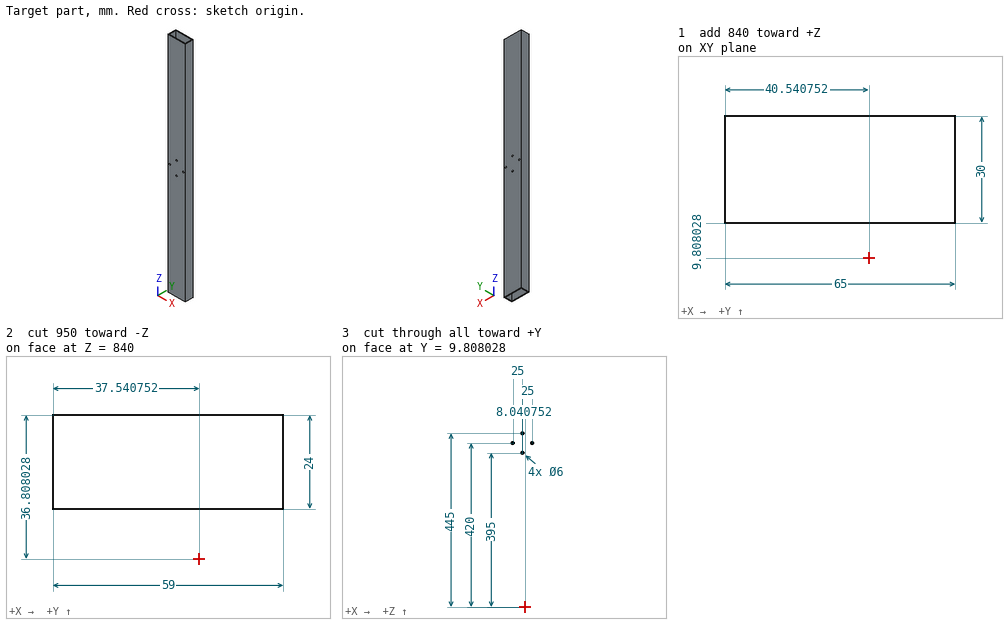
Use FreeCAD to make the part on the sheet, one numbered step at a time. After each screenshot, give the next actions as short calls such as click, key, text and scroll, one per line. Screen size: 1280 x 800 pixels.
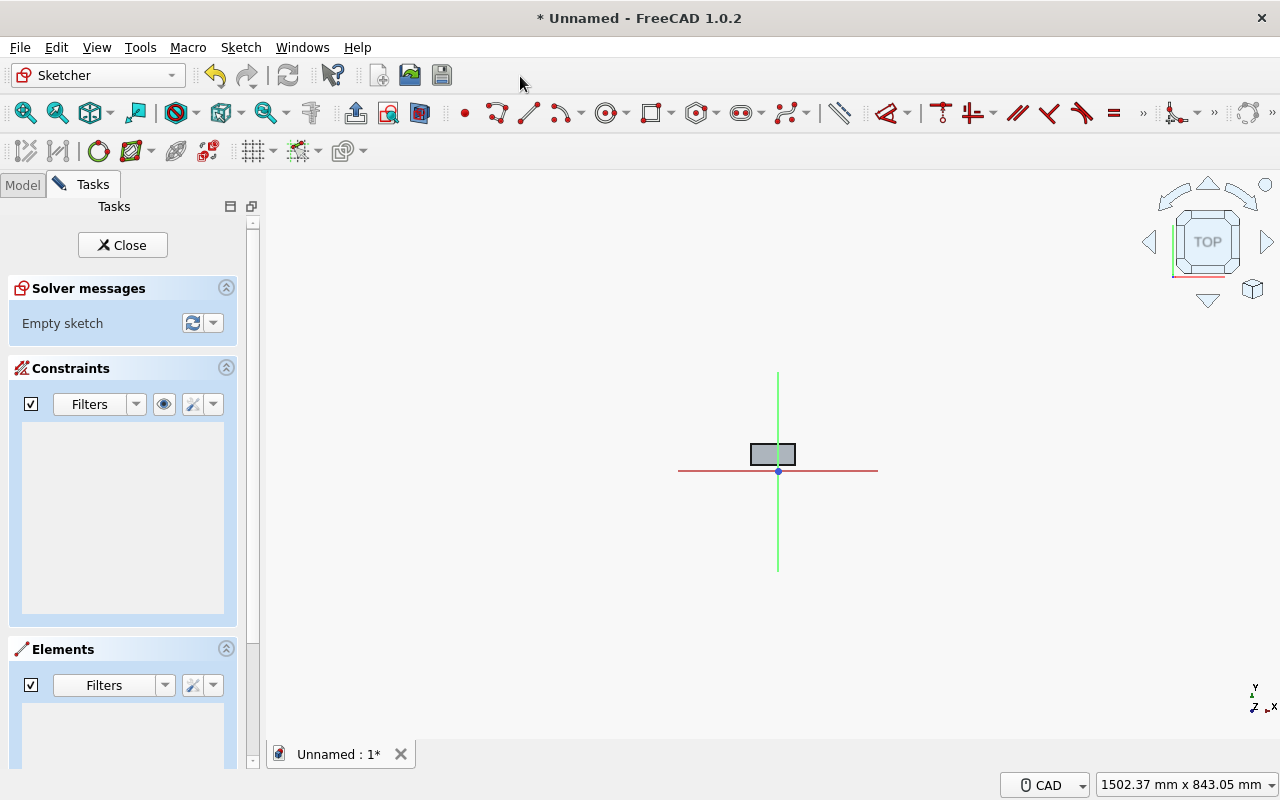
scroll(778, 459, up, 13)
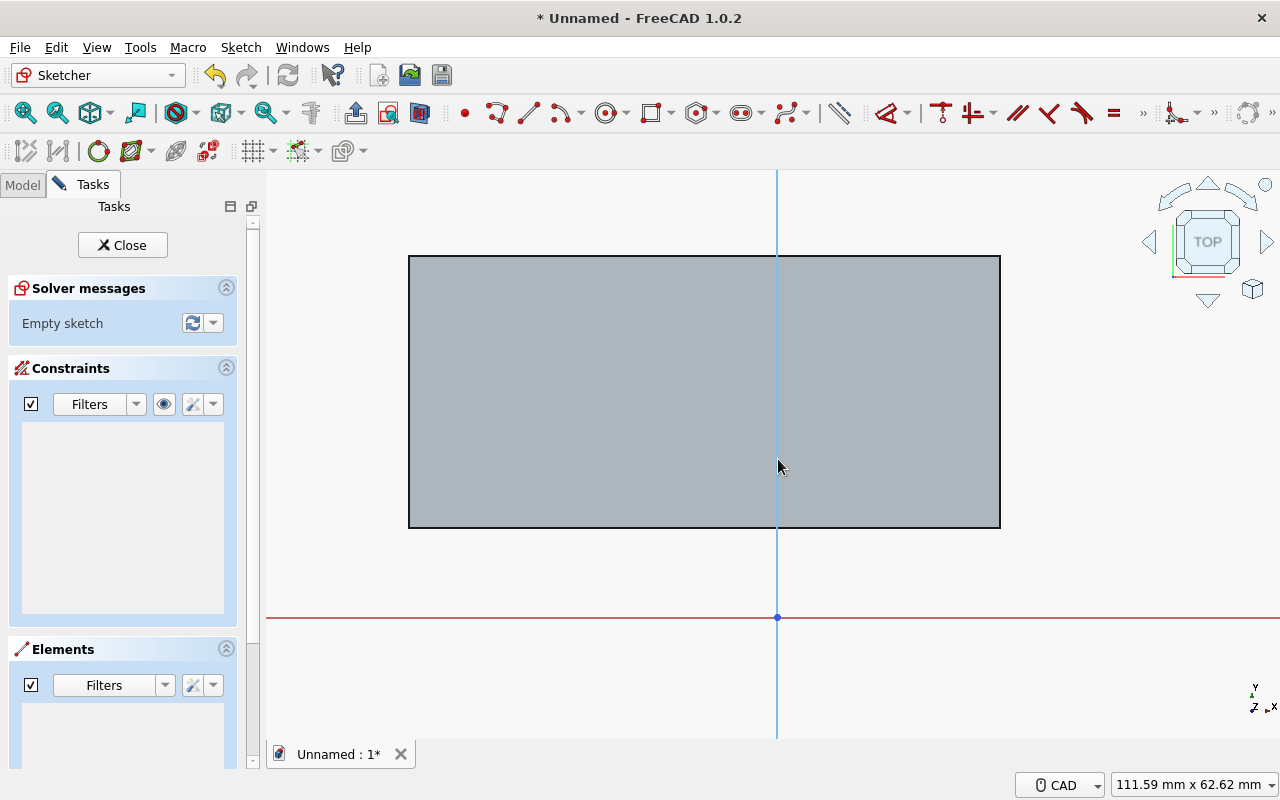
click(652, 114)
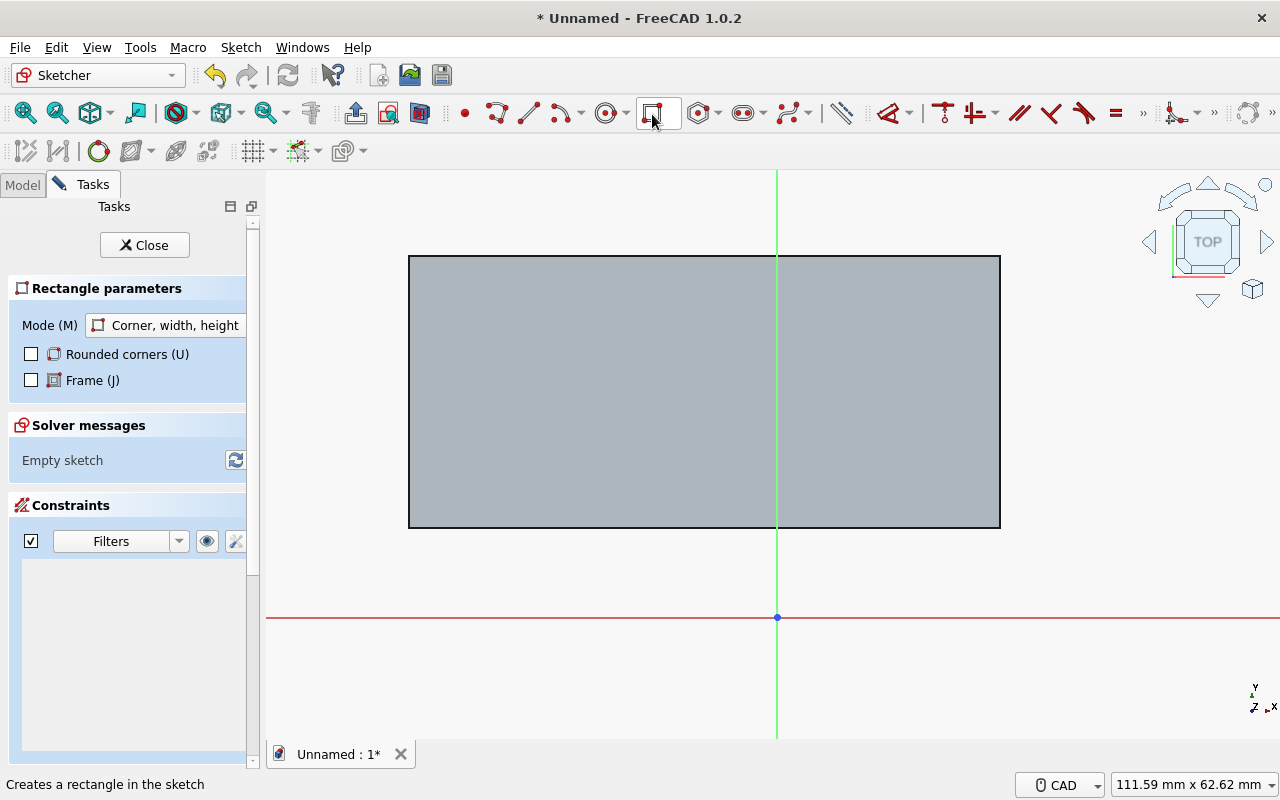
click(436, 283)
move(972, 501)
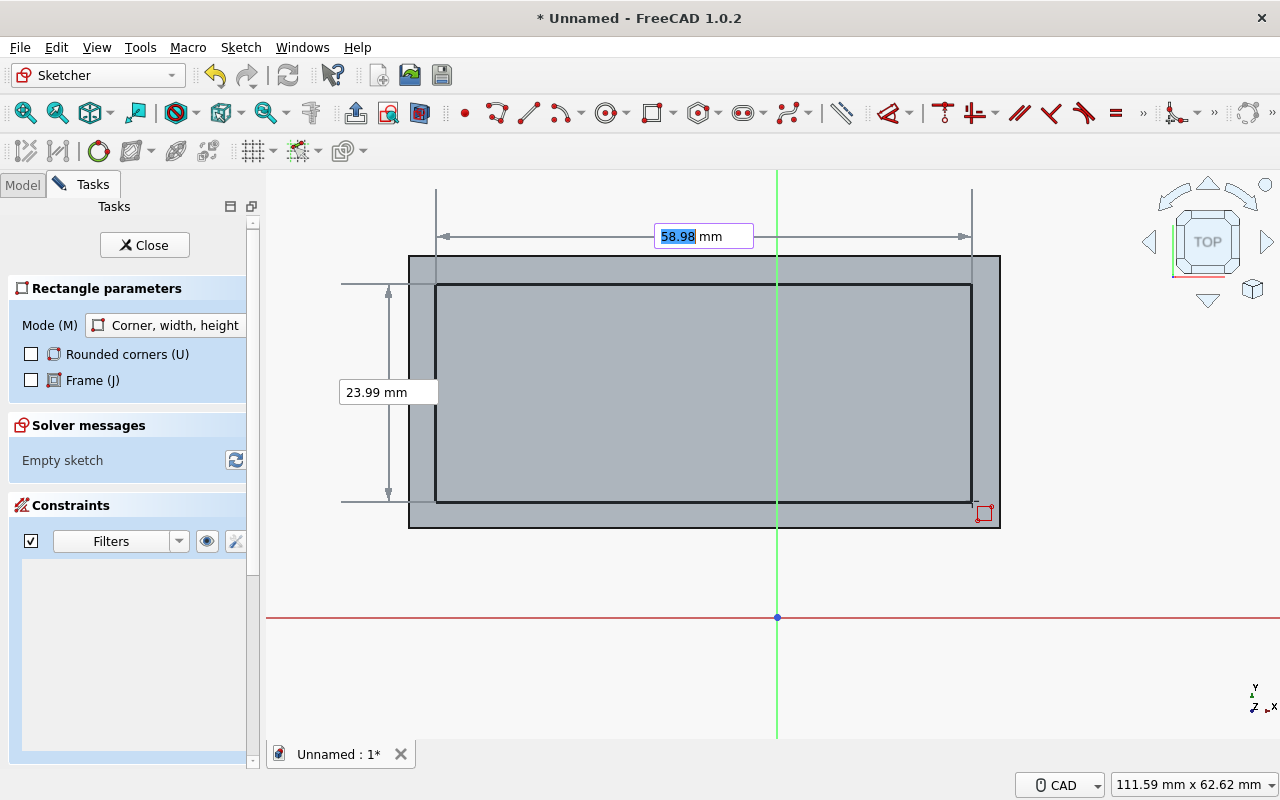
text(59)
key(Tab)
text(24)
key(Return)
key(Escape)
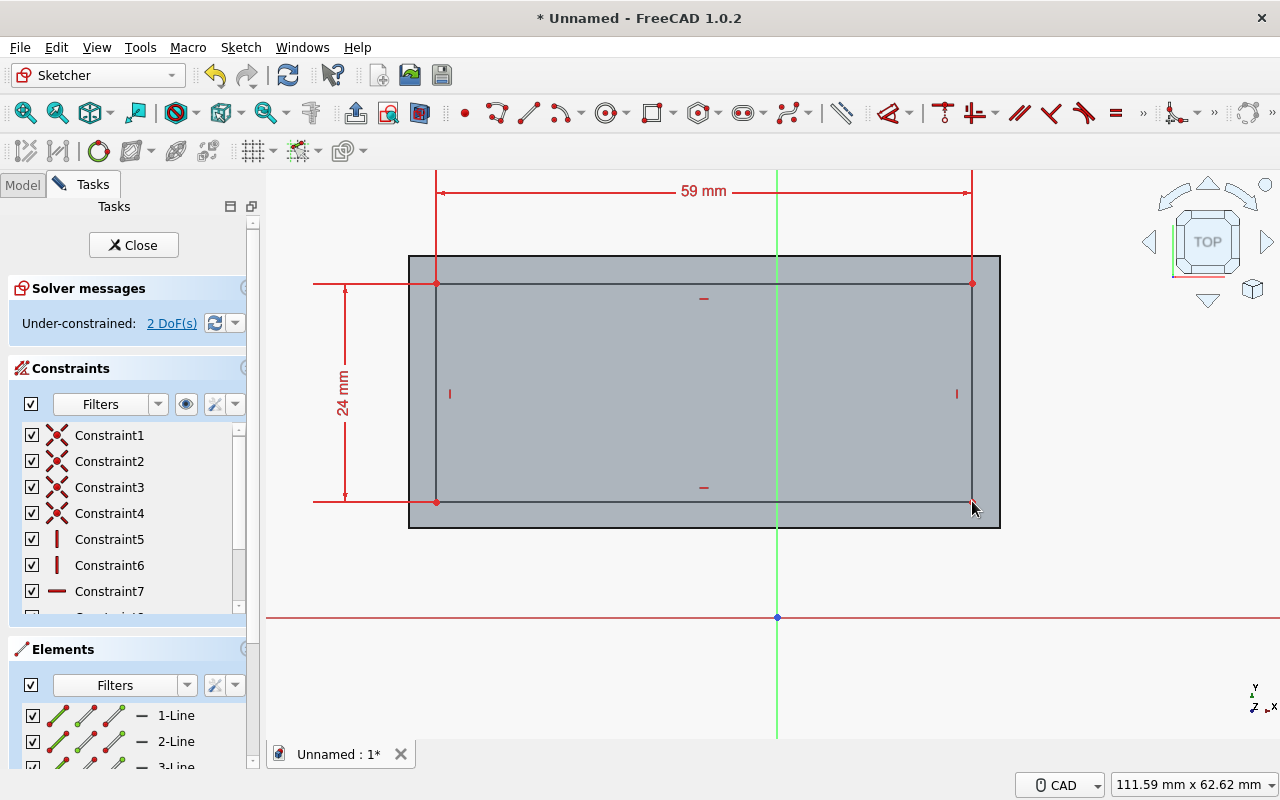
click(888, 114)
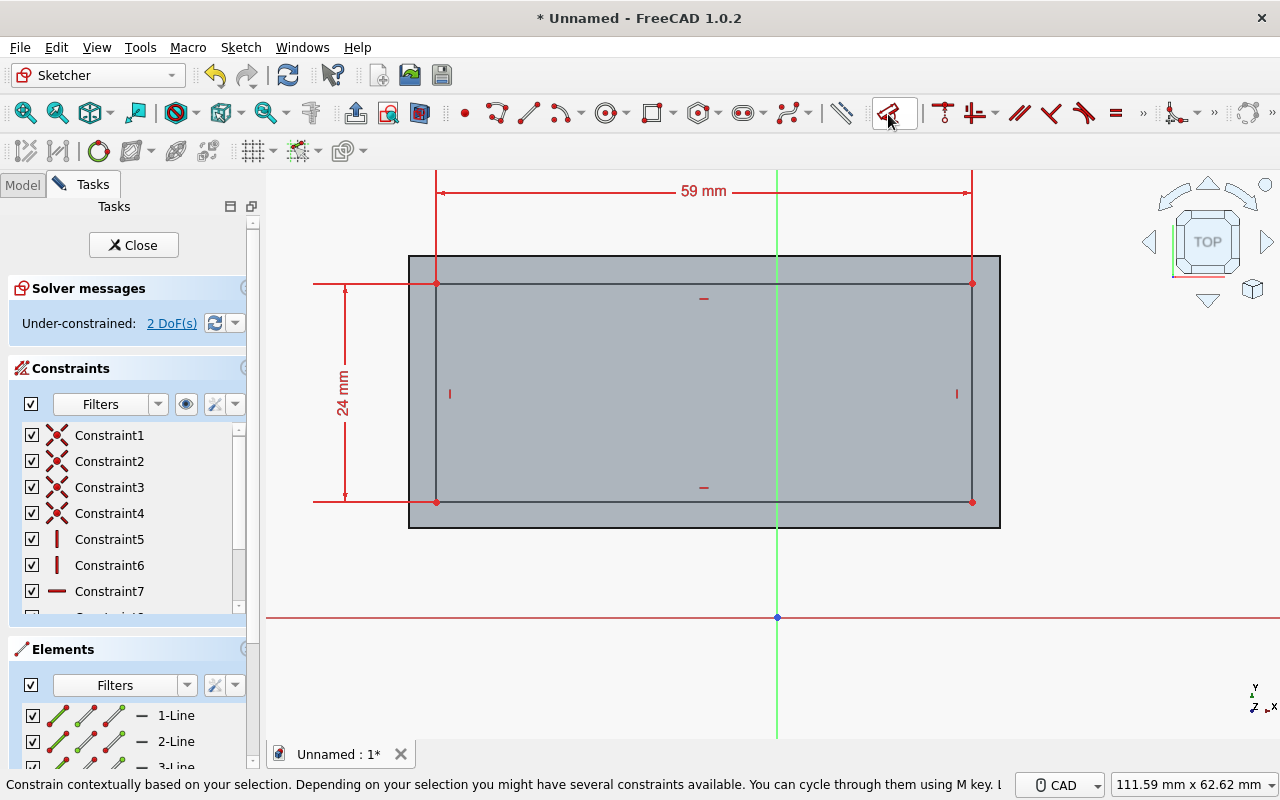
click(436, 284)
click(607, 652)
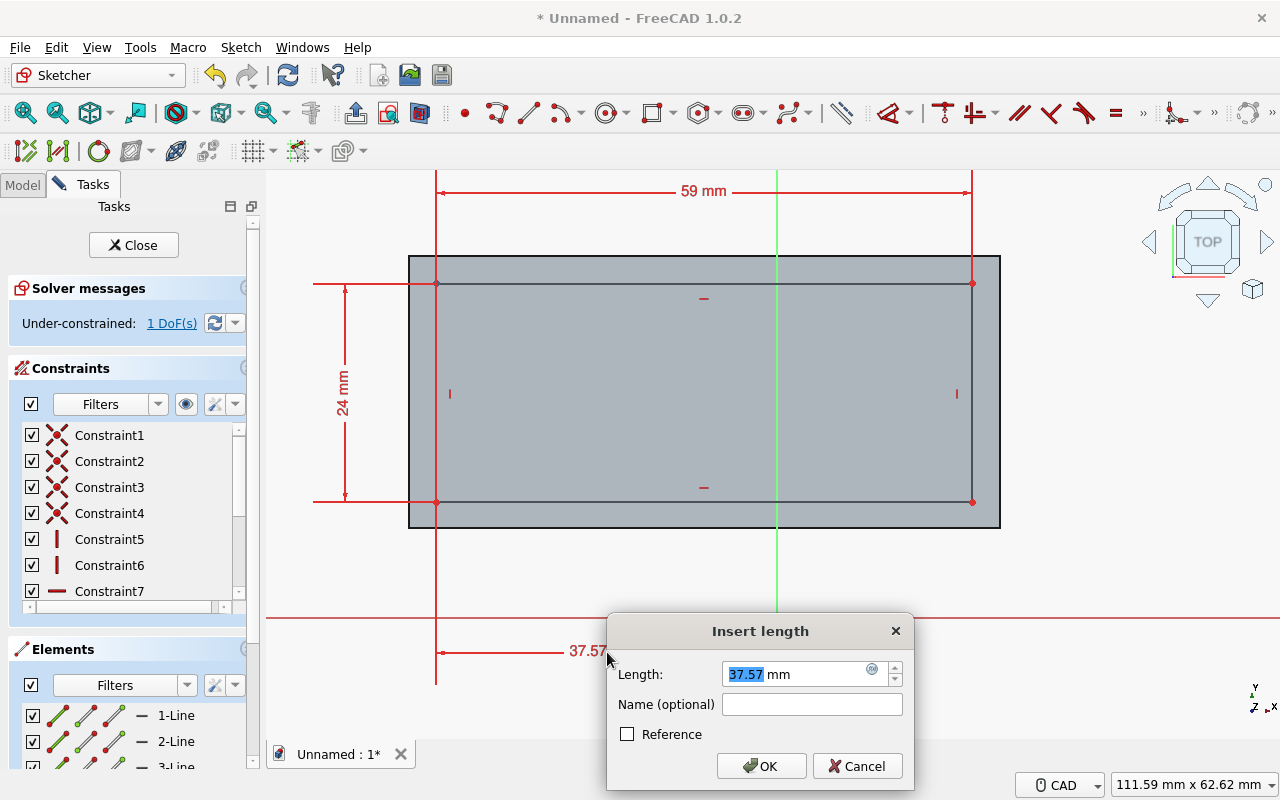
text(37.540752)
key(Return)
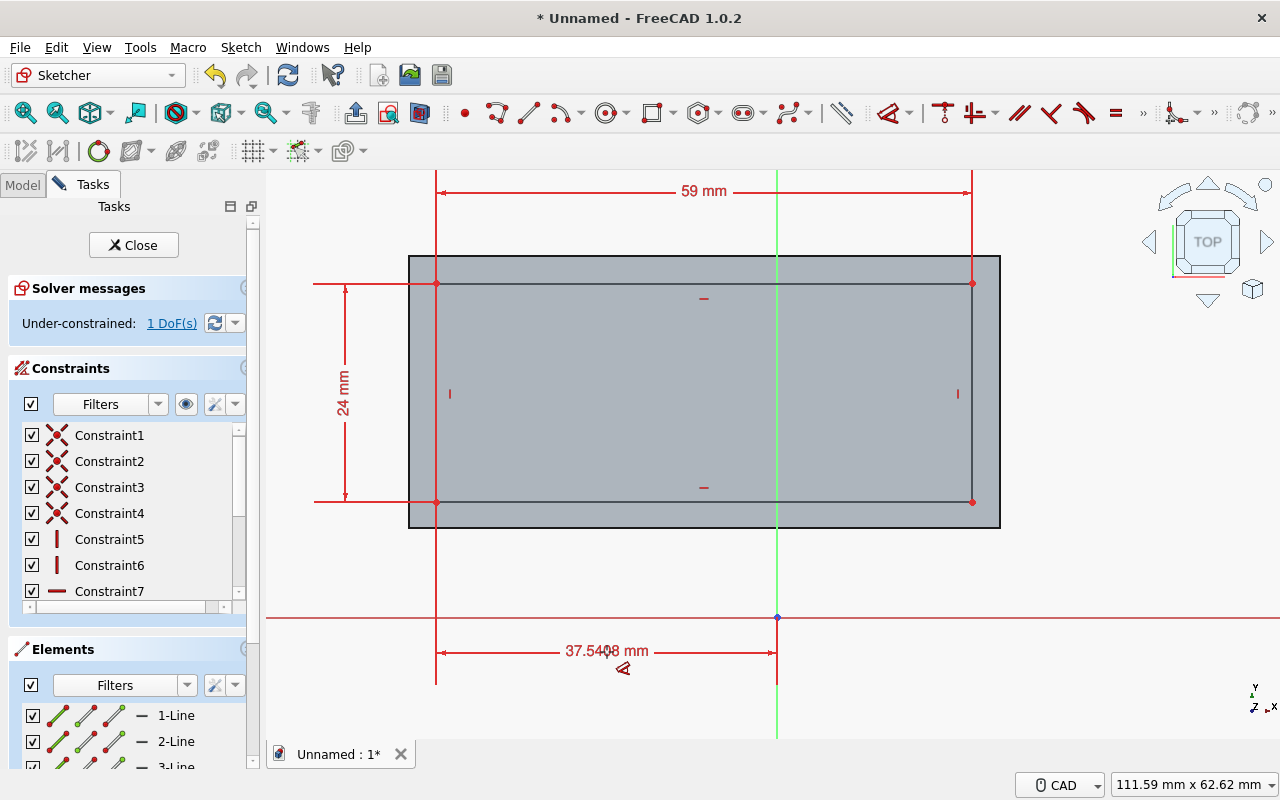
click(436, 284)
click(402, 451)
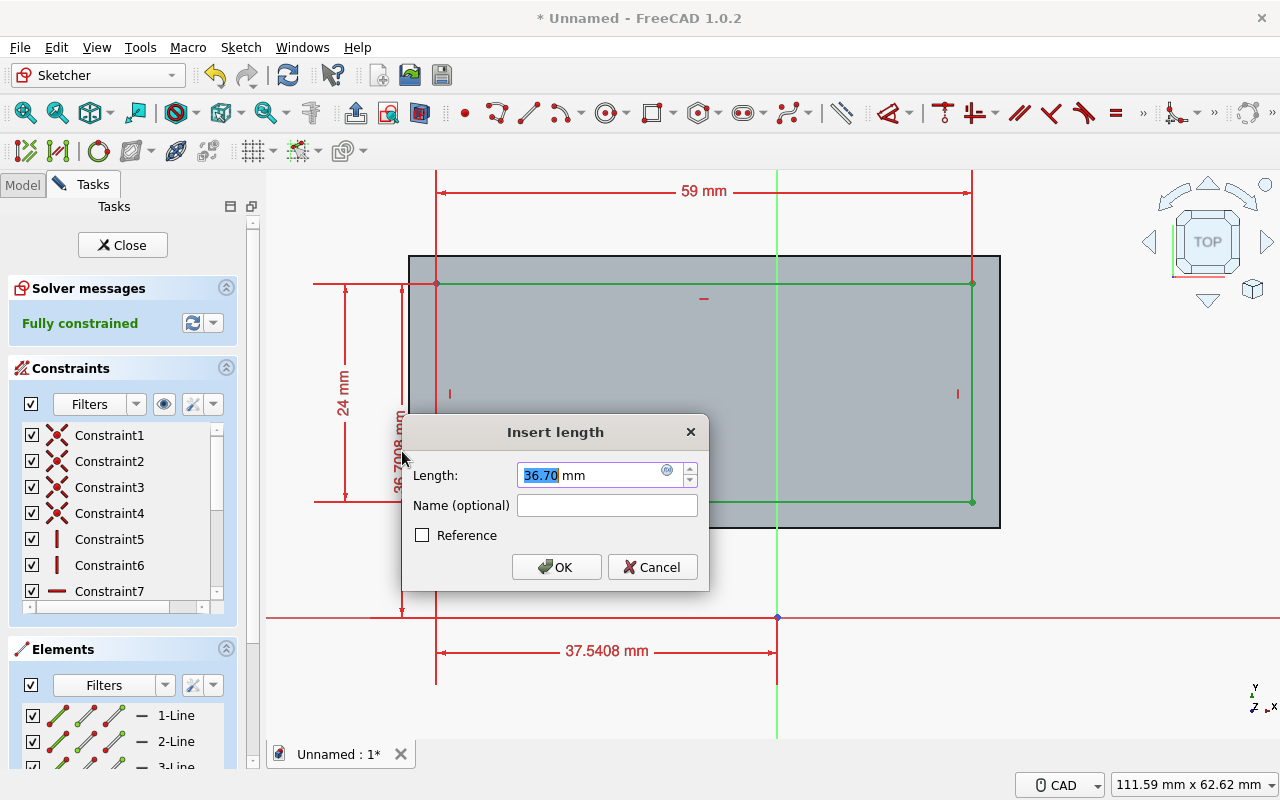
text(36.808028)
key(Return)
key(Escape)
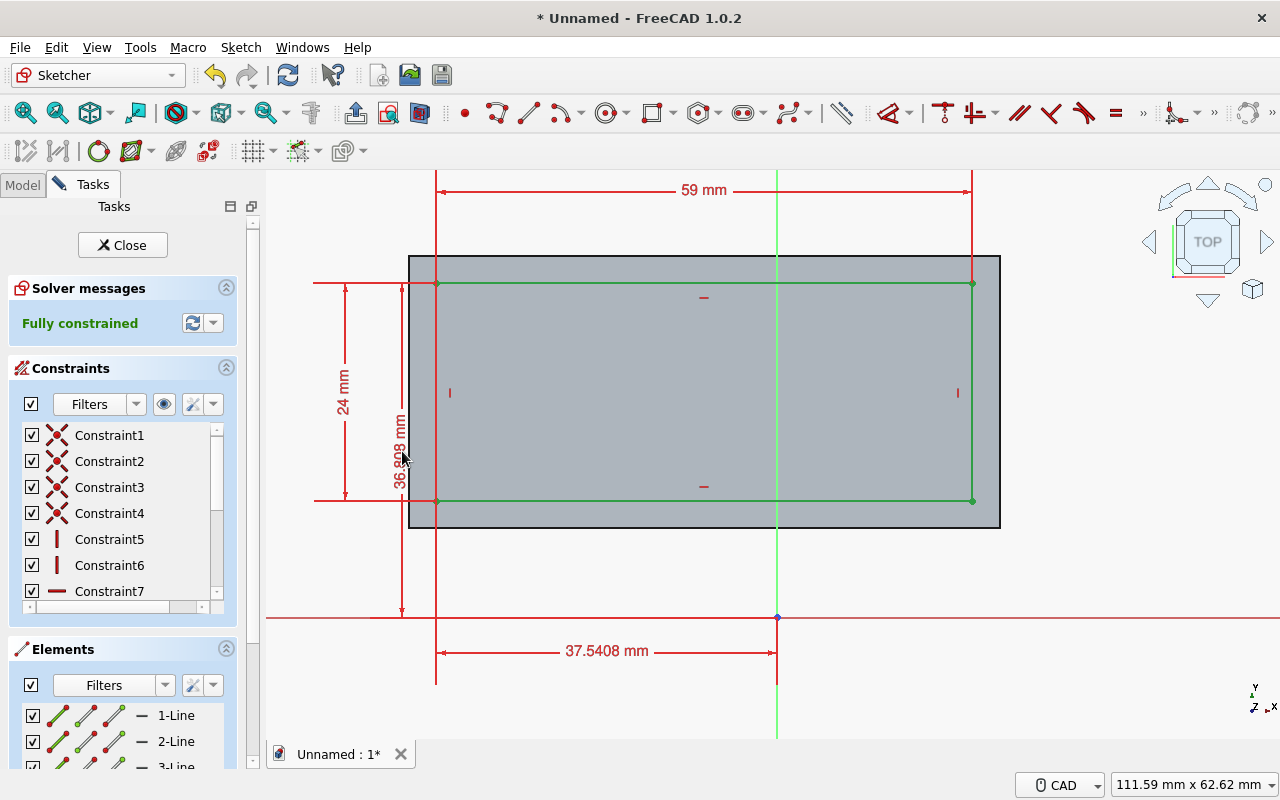
click(123, 245)